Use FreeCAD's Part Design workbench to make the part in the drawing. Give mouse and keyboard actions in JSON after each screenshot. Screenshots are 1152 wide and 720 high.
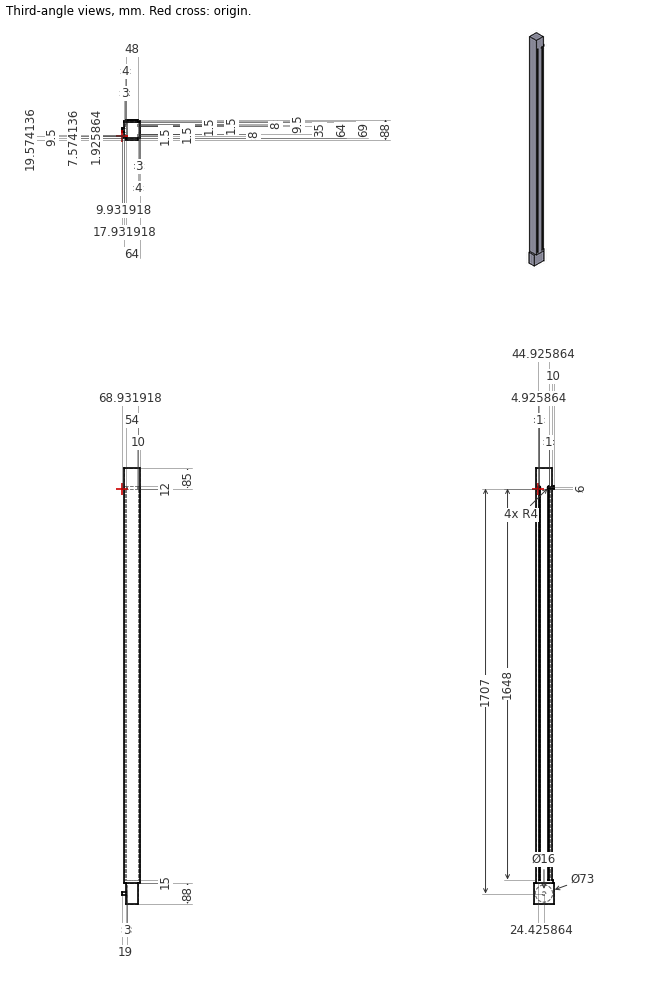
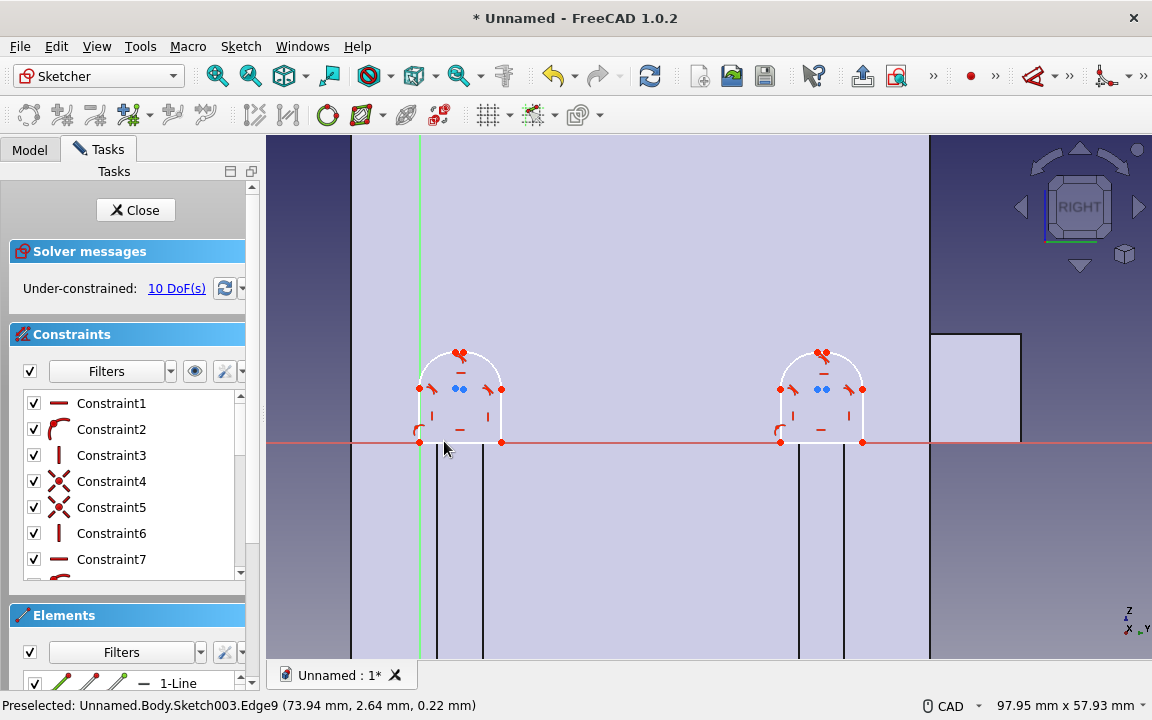
{"action": "left_click", "coordinate": [801, 357]}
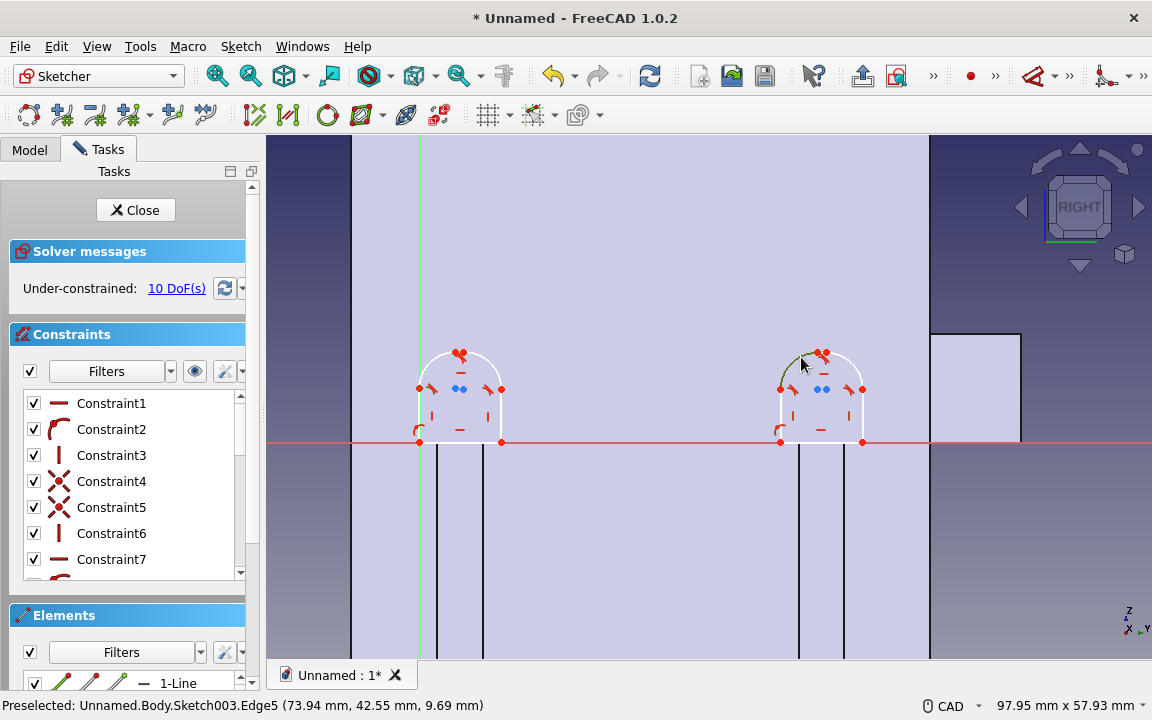
{"action": "left_click", "coordinate": [859, 373]}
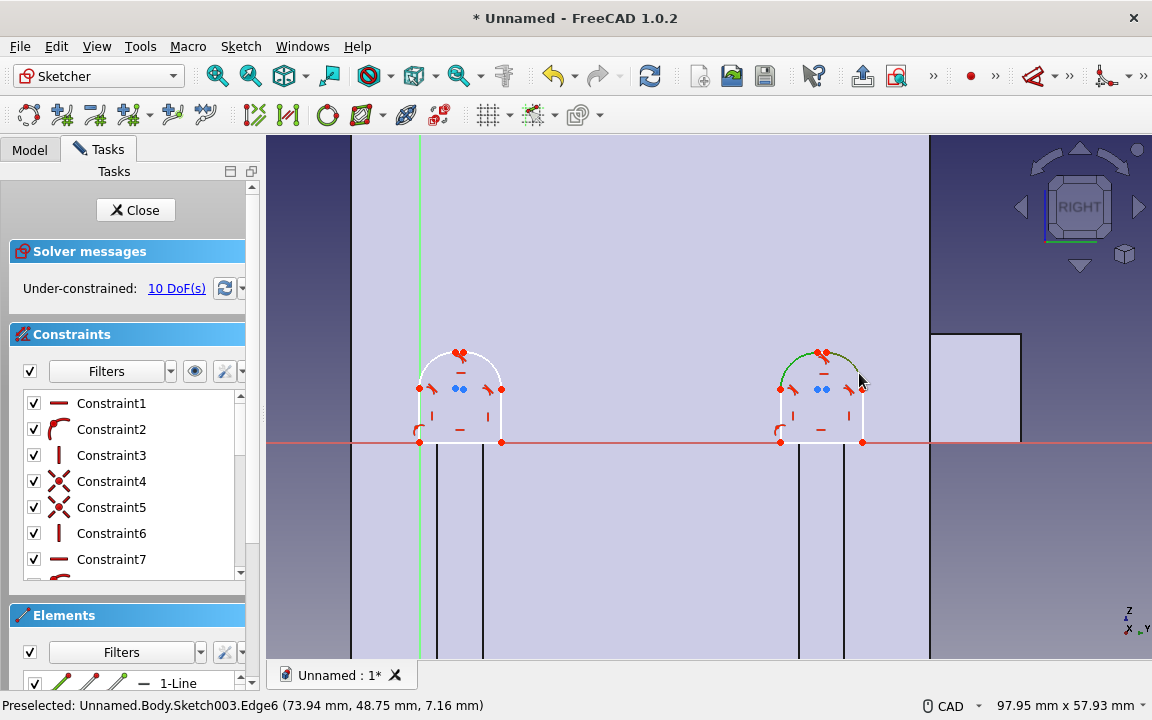
{"action": "left_click", "coordinate": [439, 356]}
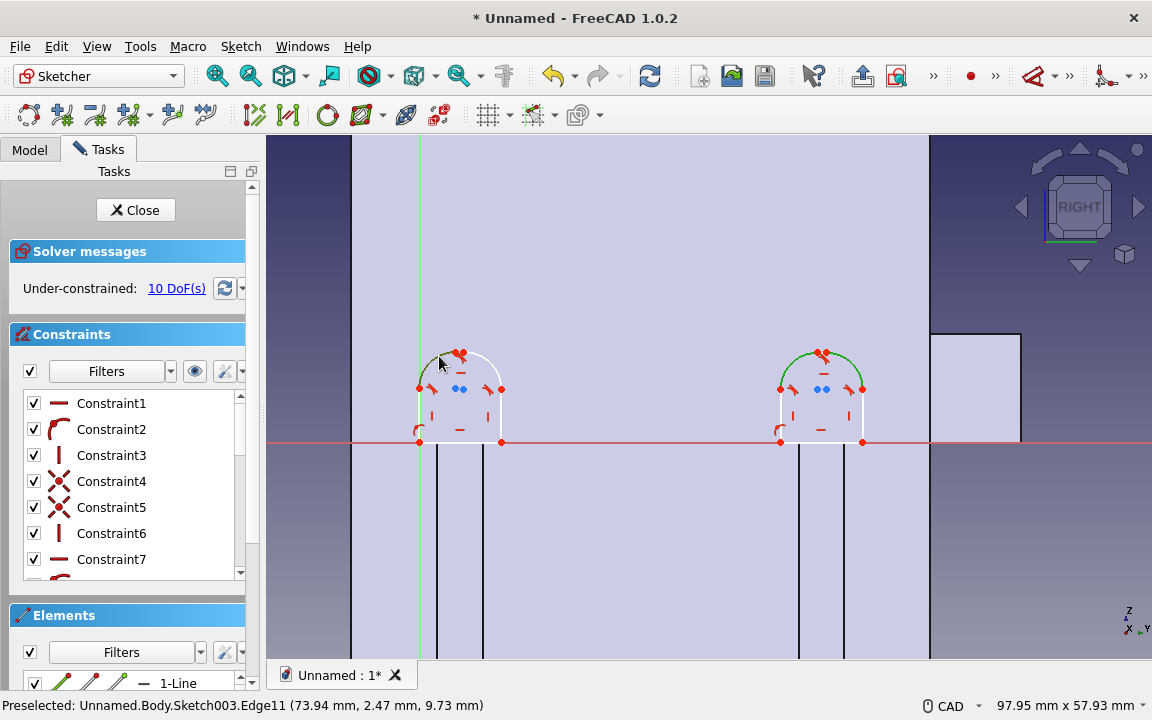
{"action": "left_click", "coordinate": [497, 372]}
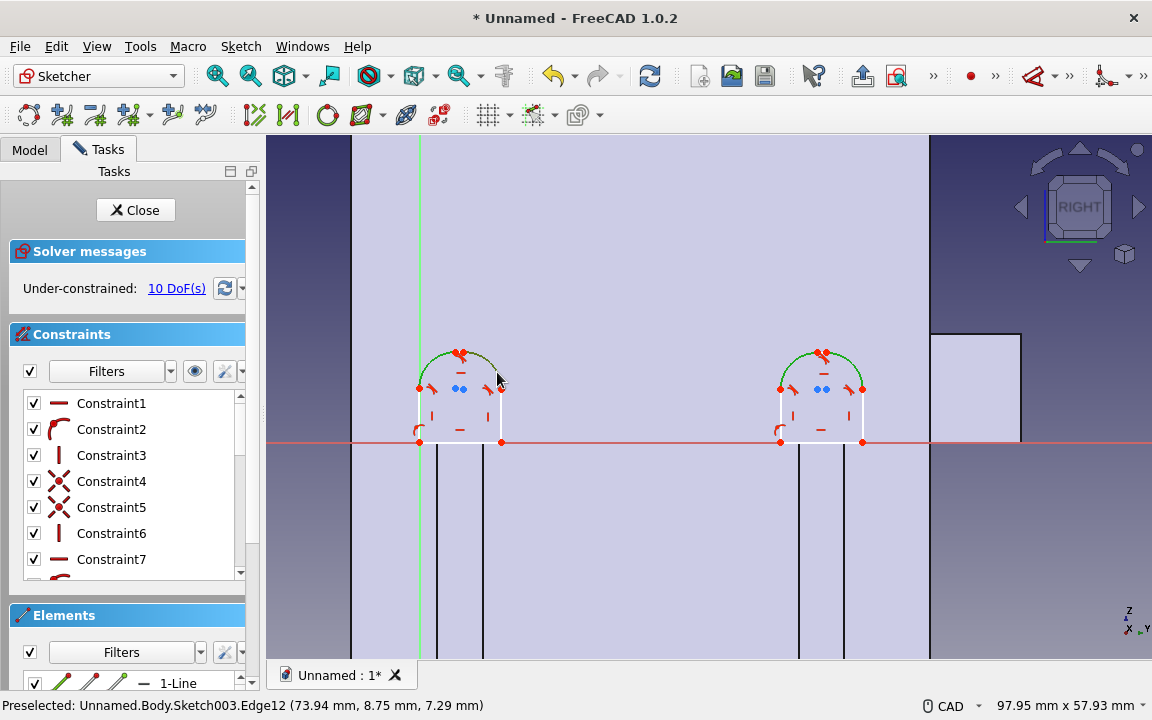
{"action": "key", "text": "e"}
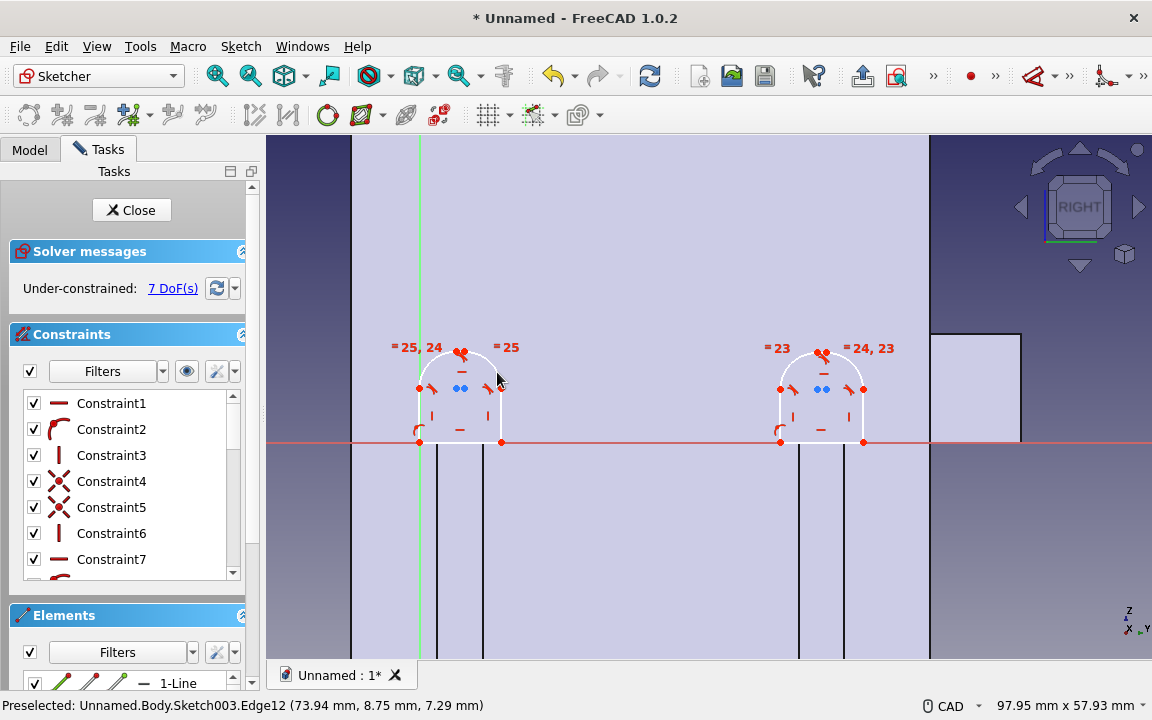
{"action": "left_click", "coordinate": [1032, 76]}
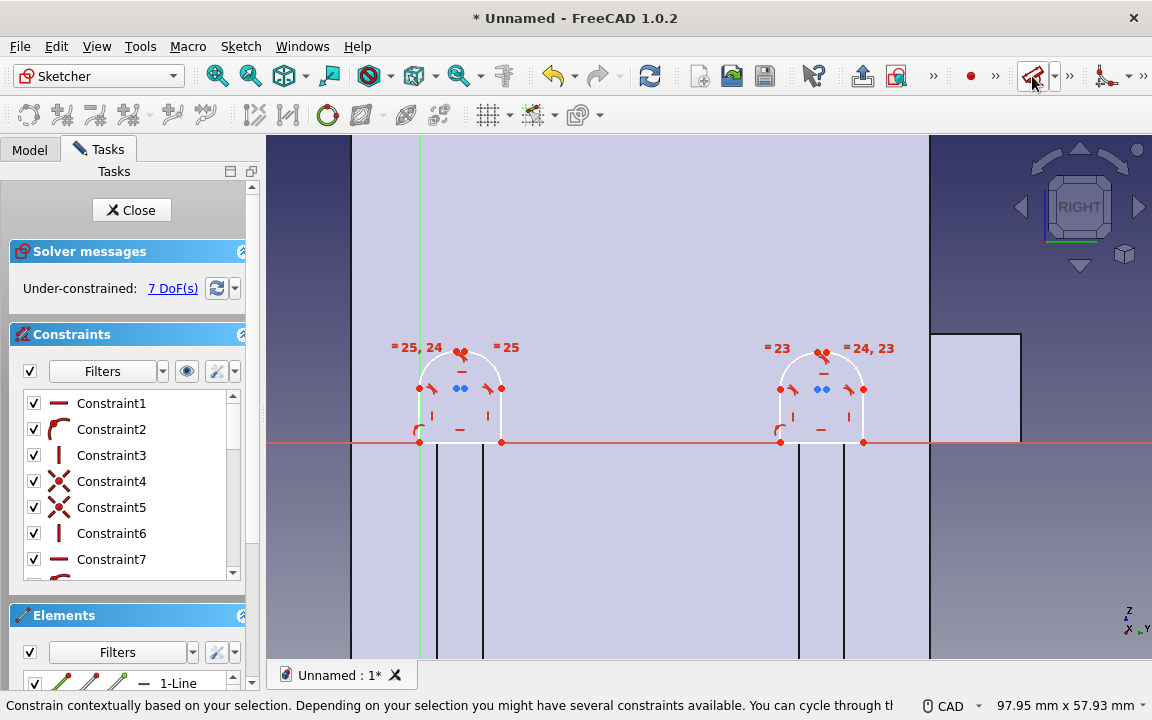
{"action": "left_click", "coordinate": [800, 357]}
{"action": "left_click", "coordinate": [785, 329]}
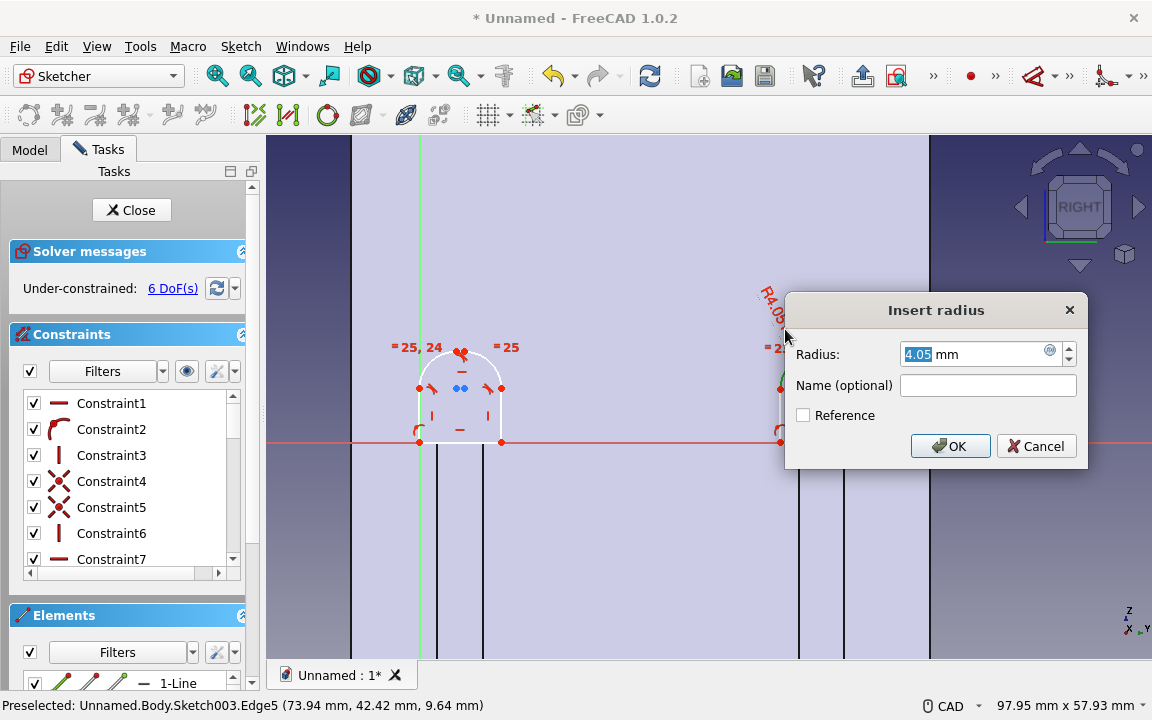
{"action": "type", "text": "4"}
{"action": "key", "text": "Return"}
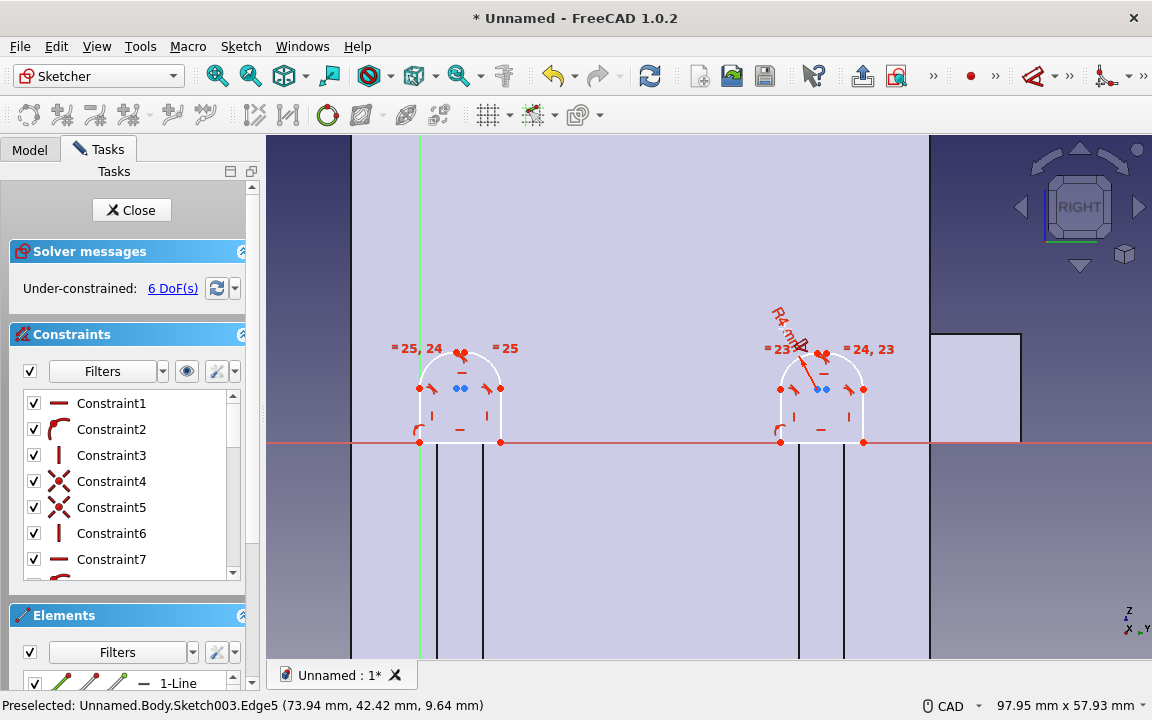
{"action": "scroll", "coordinate": [822, 353], "scroll_direction": "up", "scroll_amount": 8}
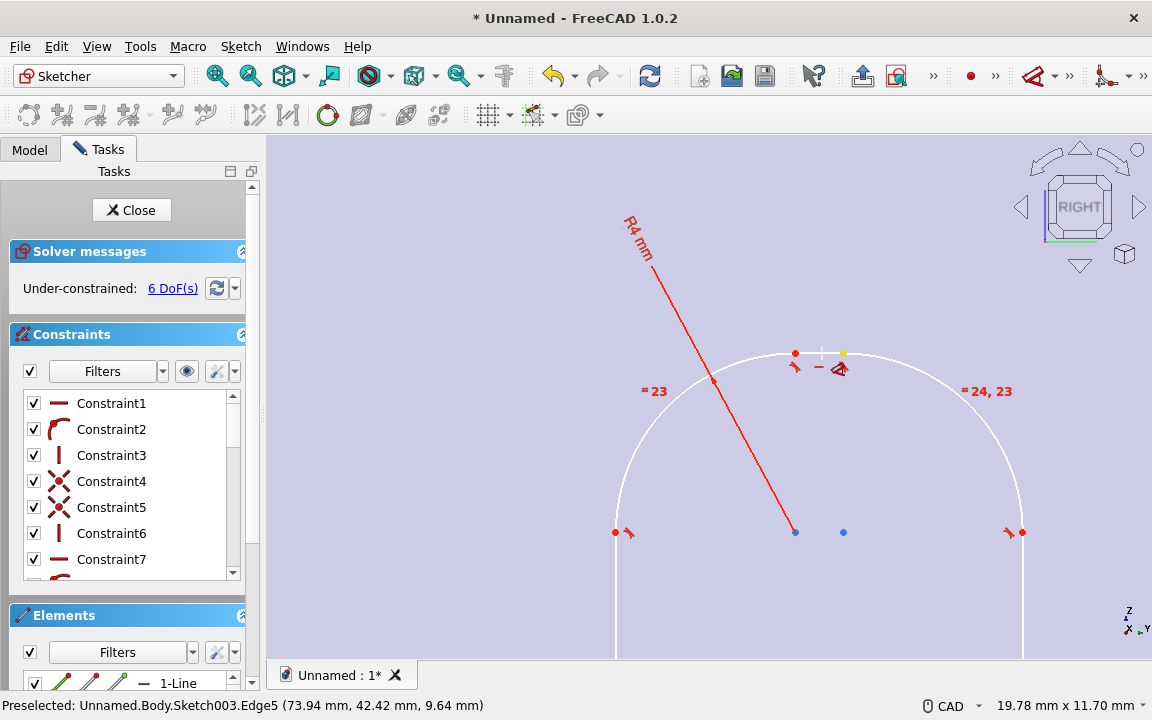
{"action": "left_click", "coordinate": [819, 353]}
{"action": "left_click", "coordinate": [819, 319]}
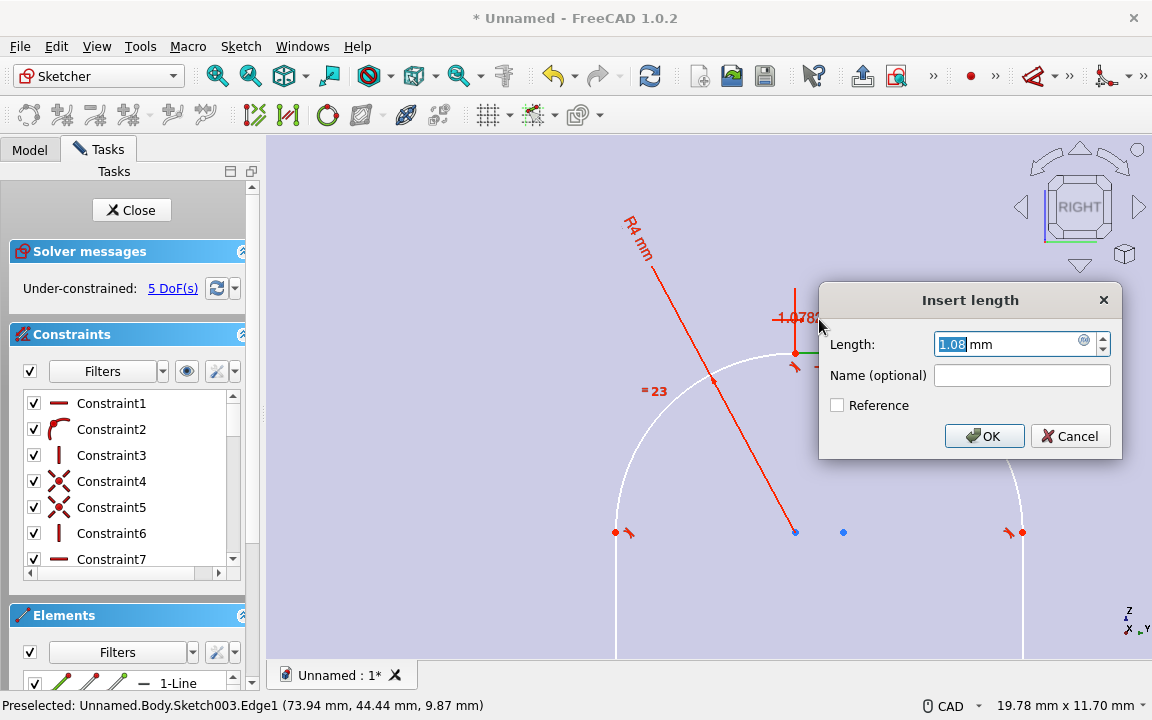
{"action": "type", "text": "1"}
{"action": "key", "text": "Return"}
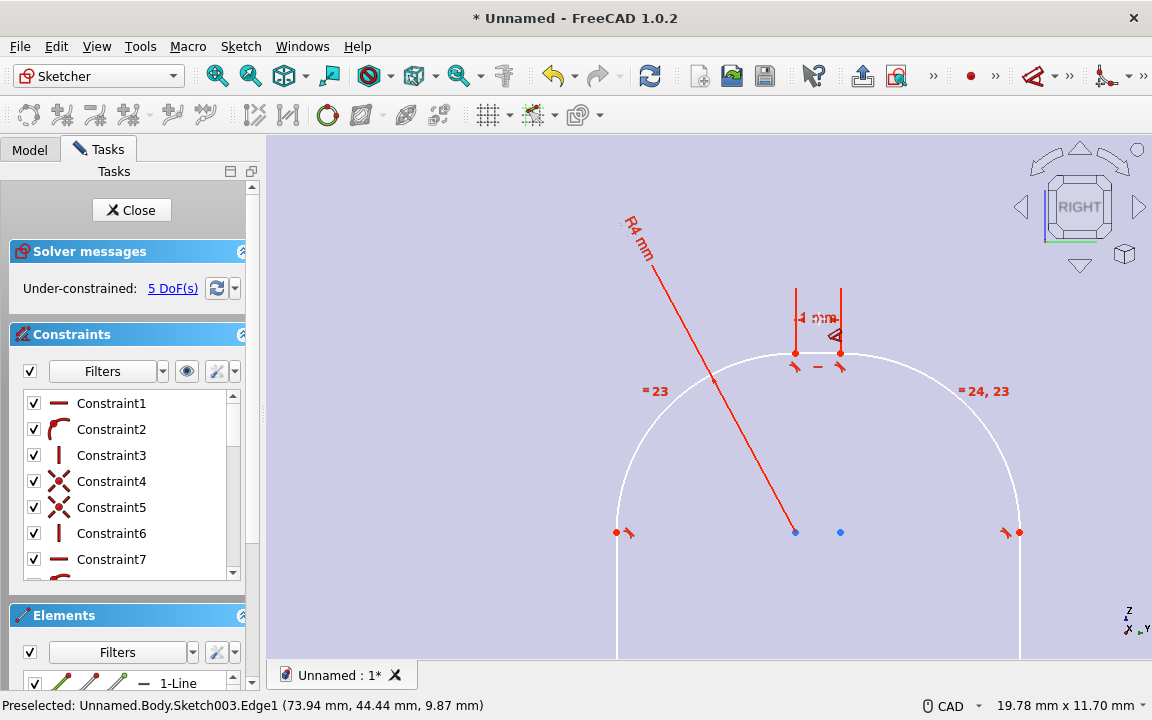
{"action": "scroll", "coordinate": [822, 353], "scroll_direction": "down", "scroll_amount": 8}